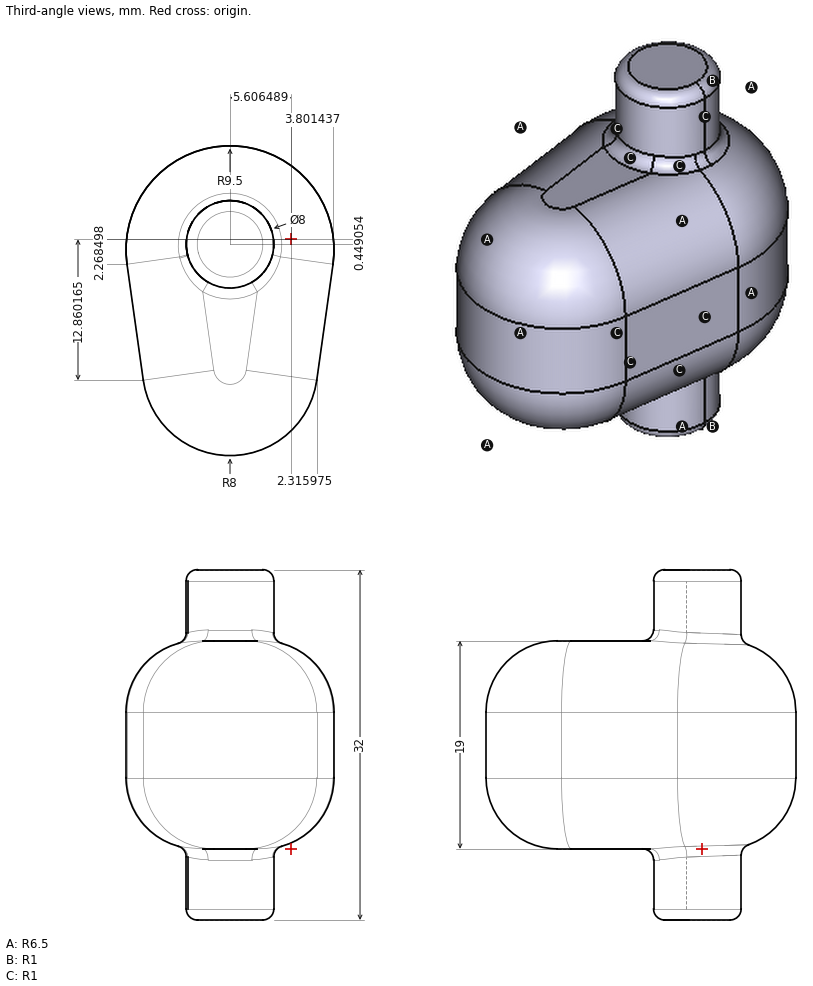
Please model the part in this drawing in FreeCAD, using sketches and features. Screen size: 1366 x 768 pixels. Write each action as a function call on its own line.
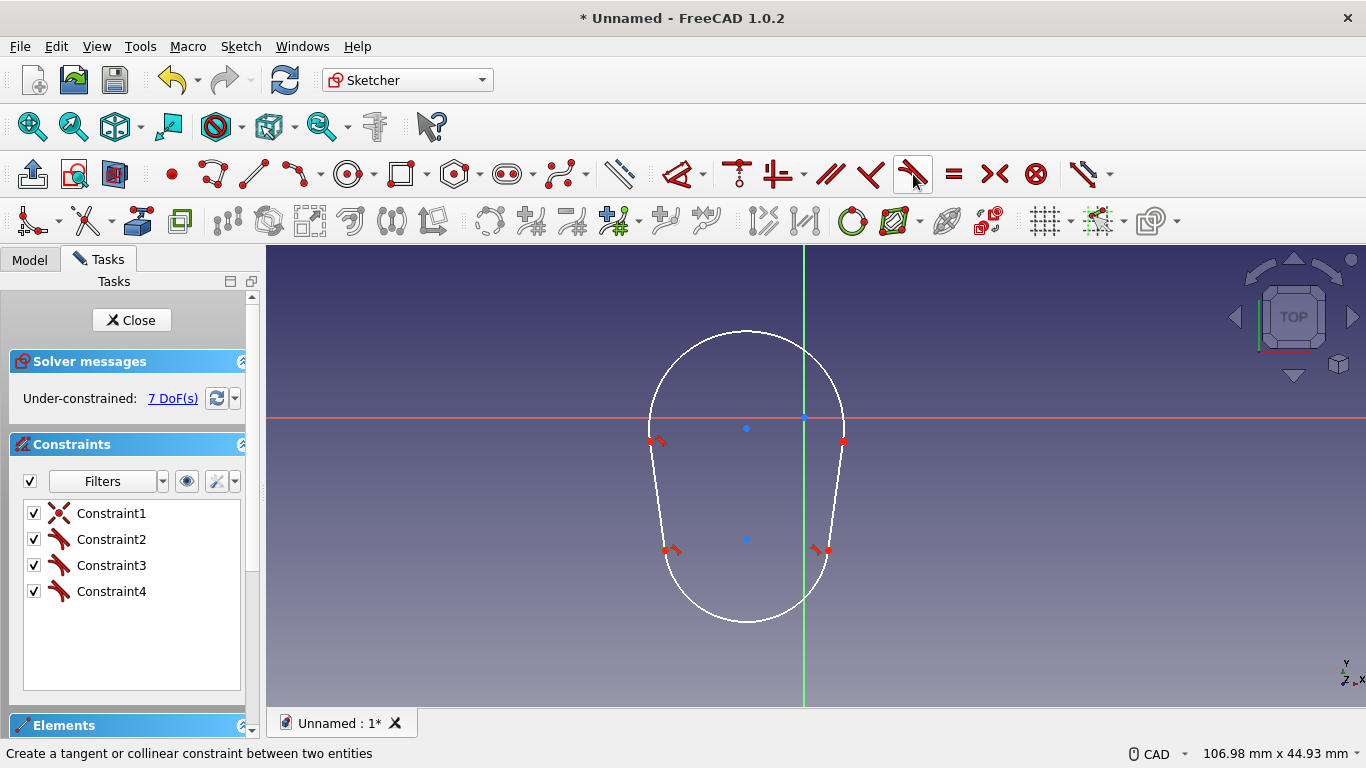
click(832, 518)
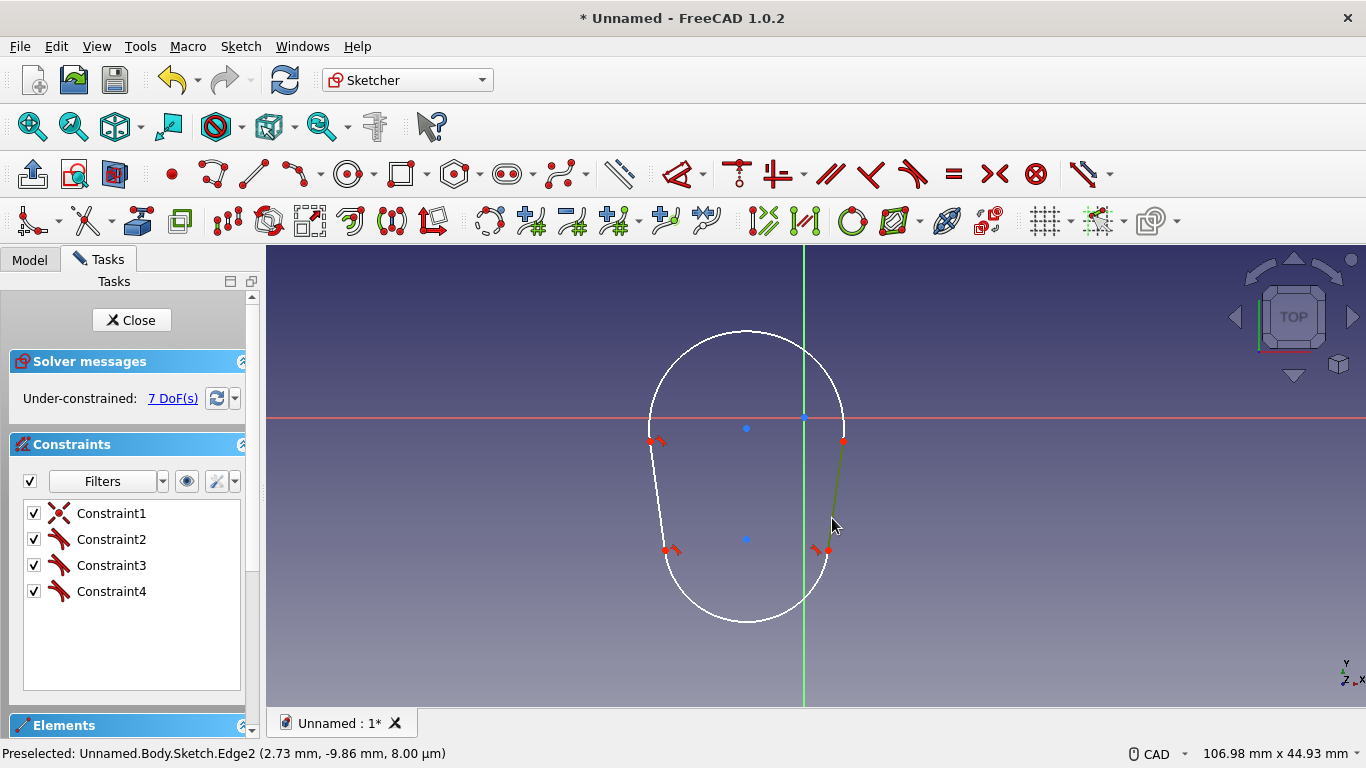
click(808, 353)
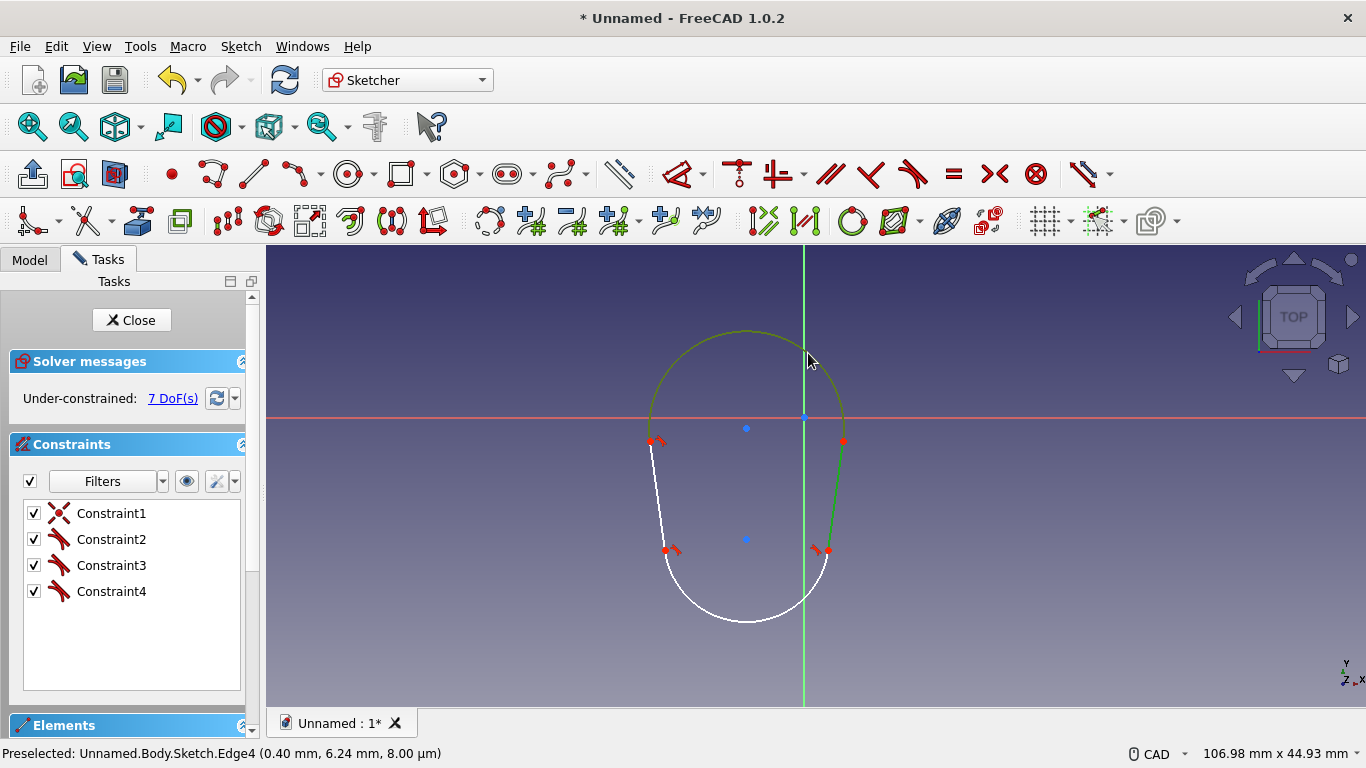
key(t)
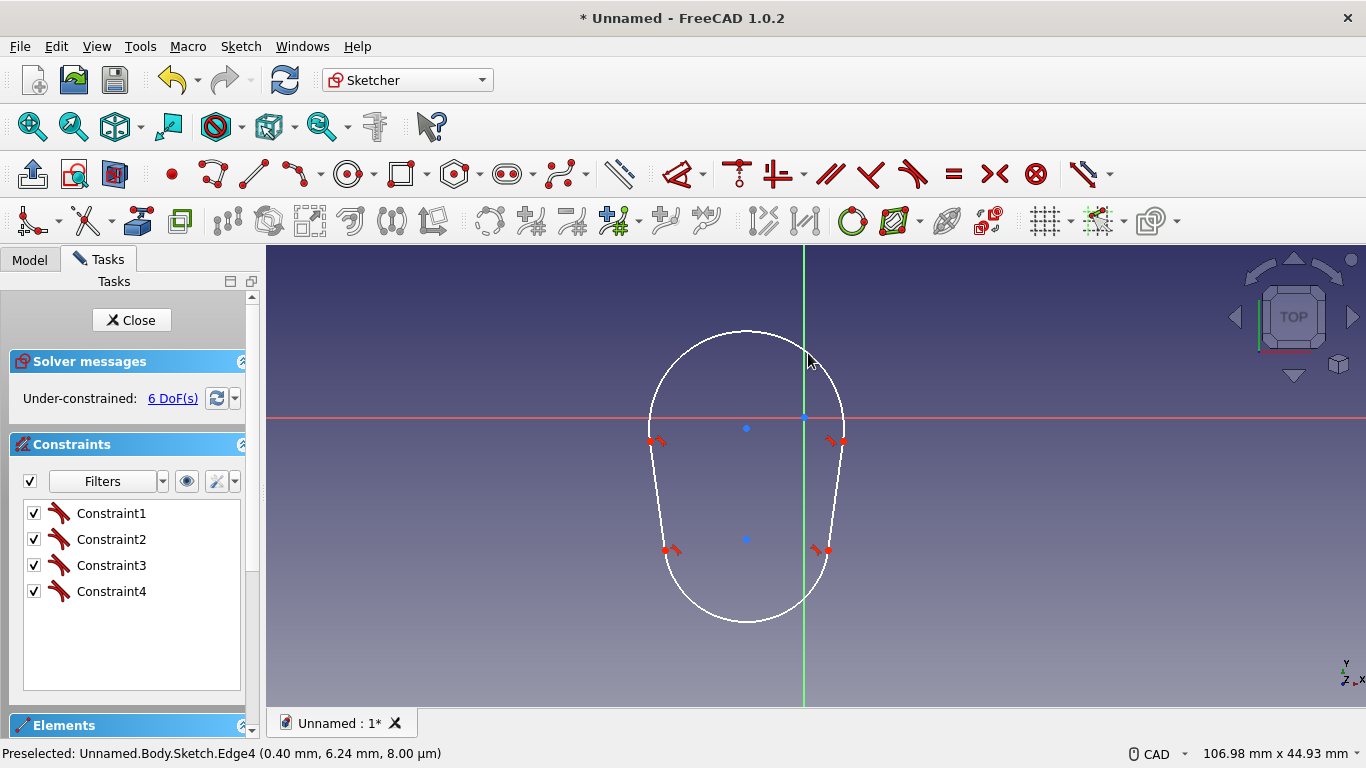
click(702, 609)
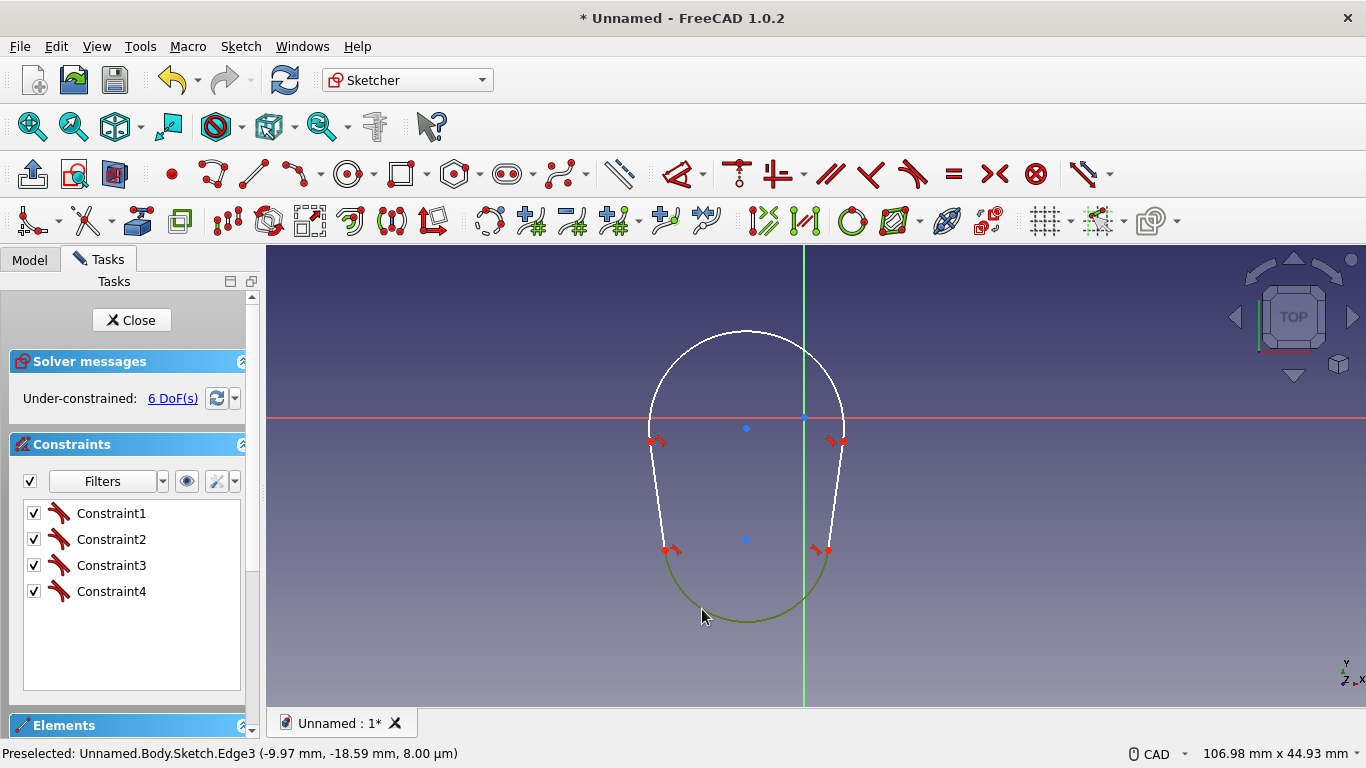
key(k)
key(r)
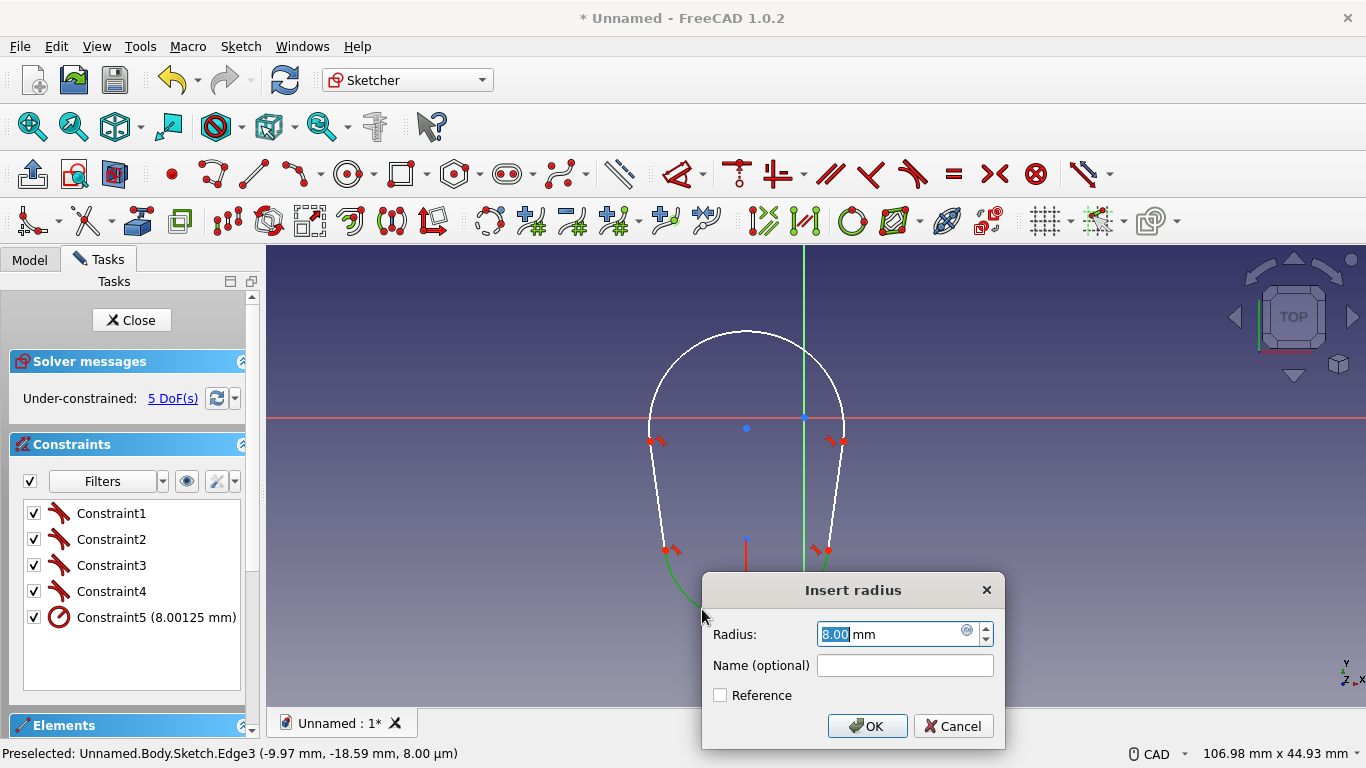
text(8)
key(Return)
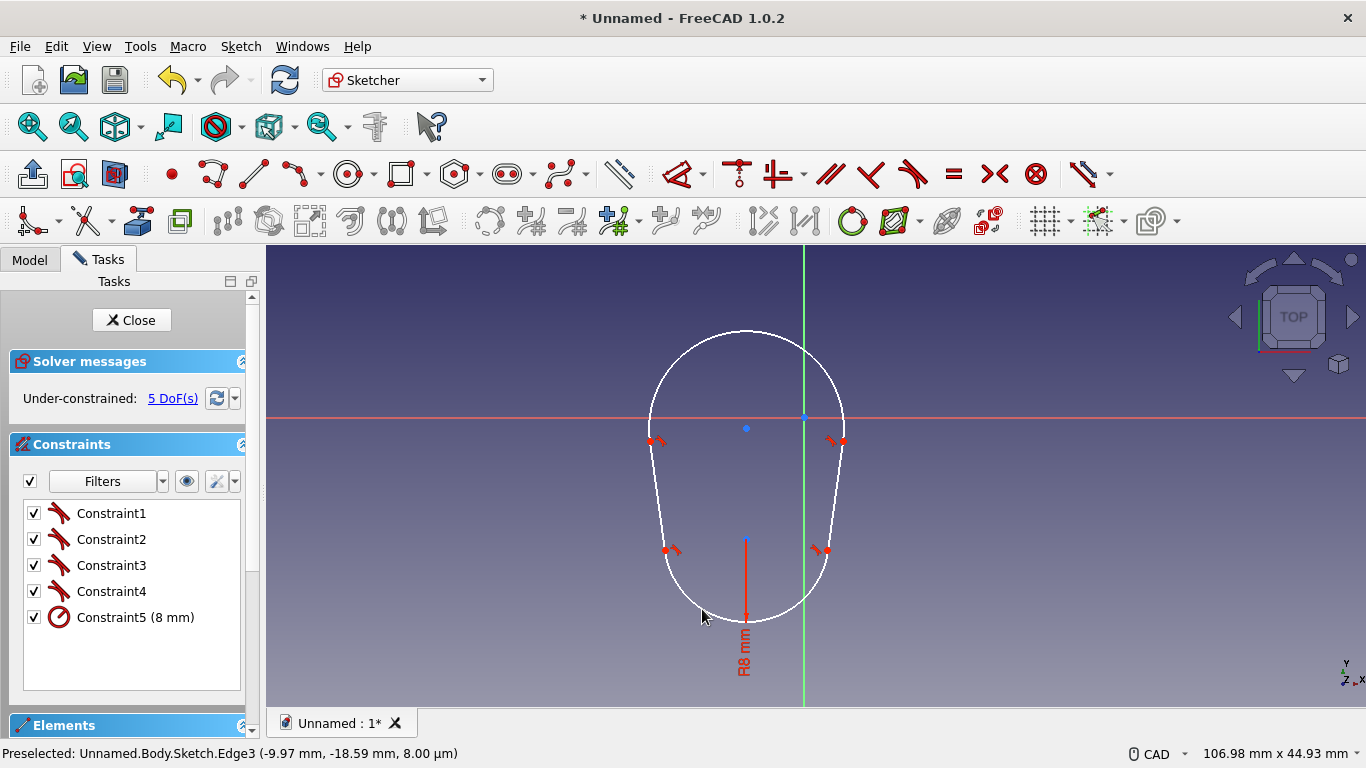
click(808, 353)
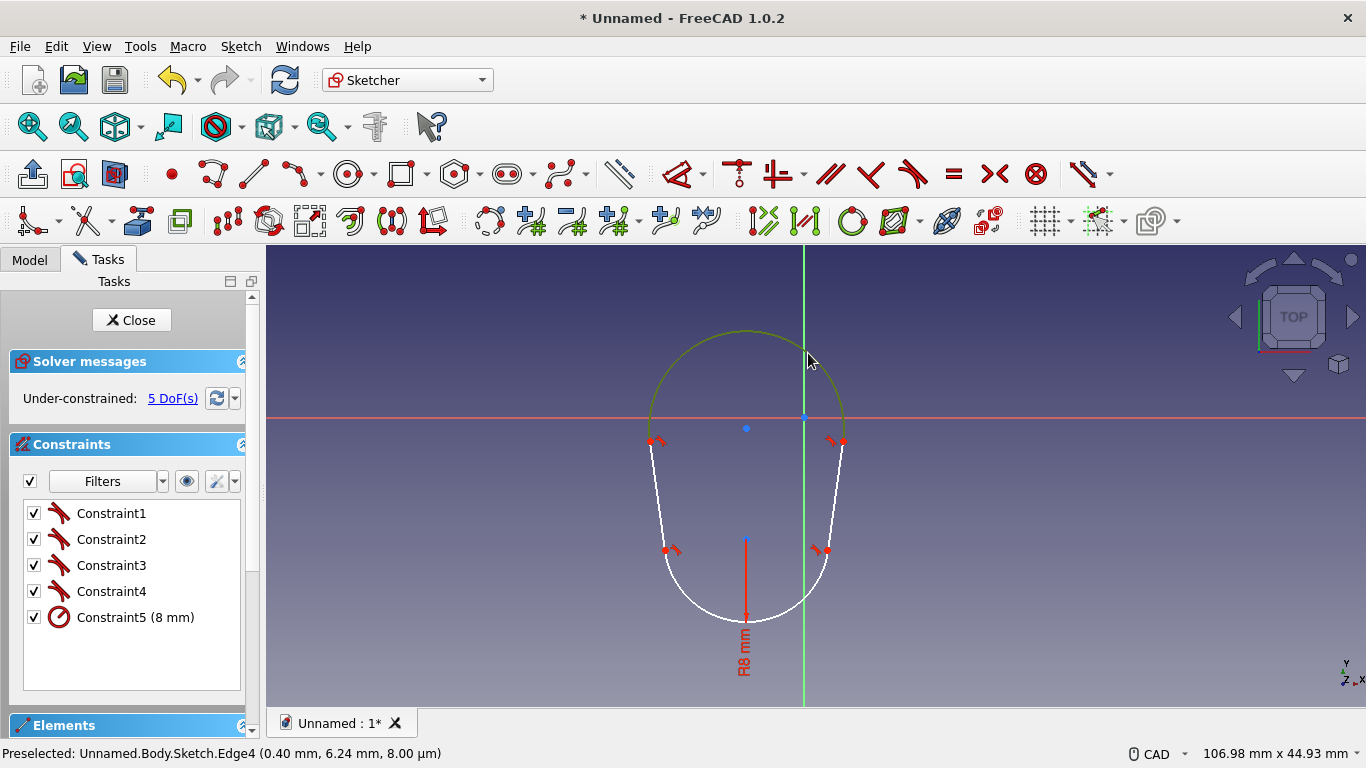
key(k)
key(r)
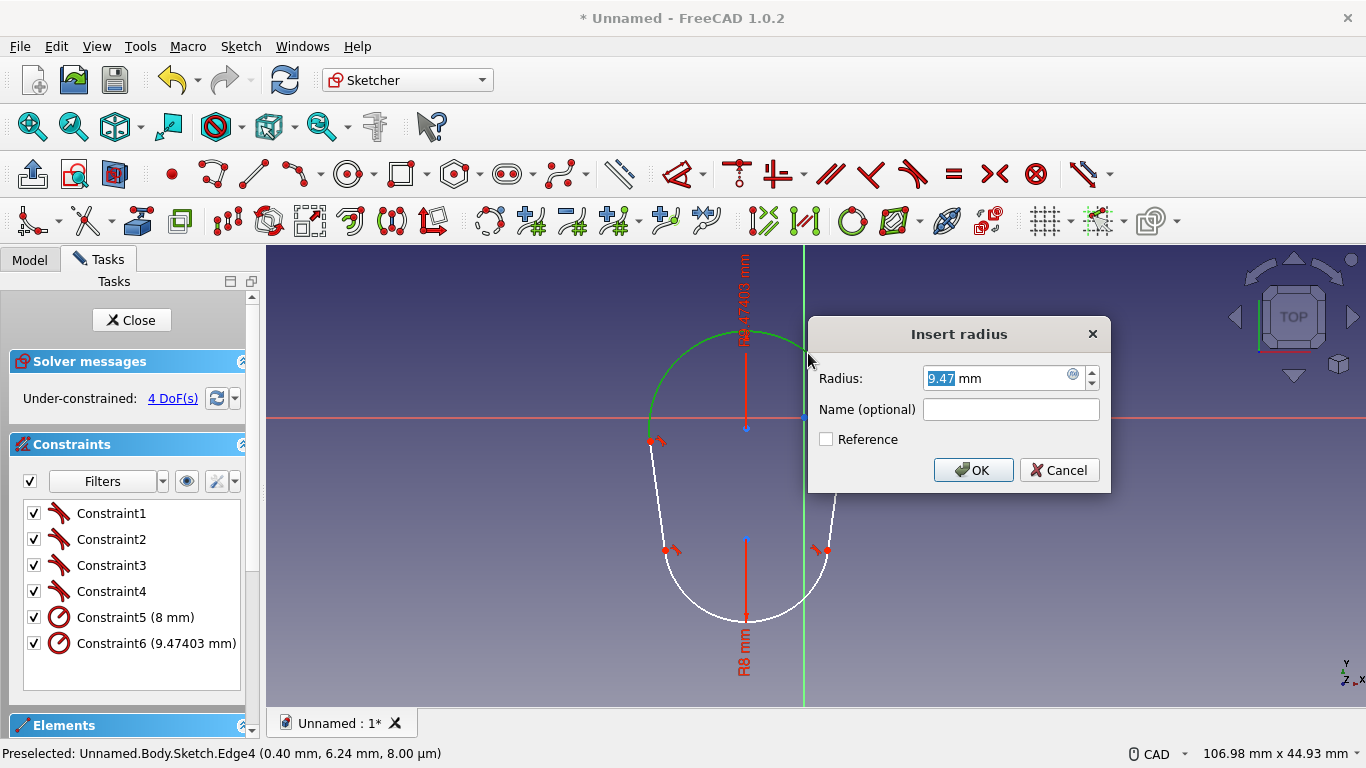
text(9.5)
key(Return)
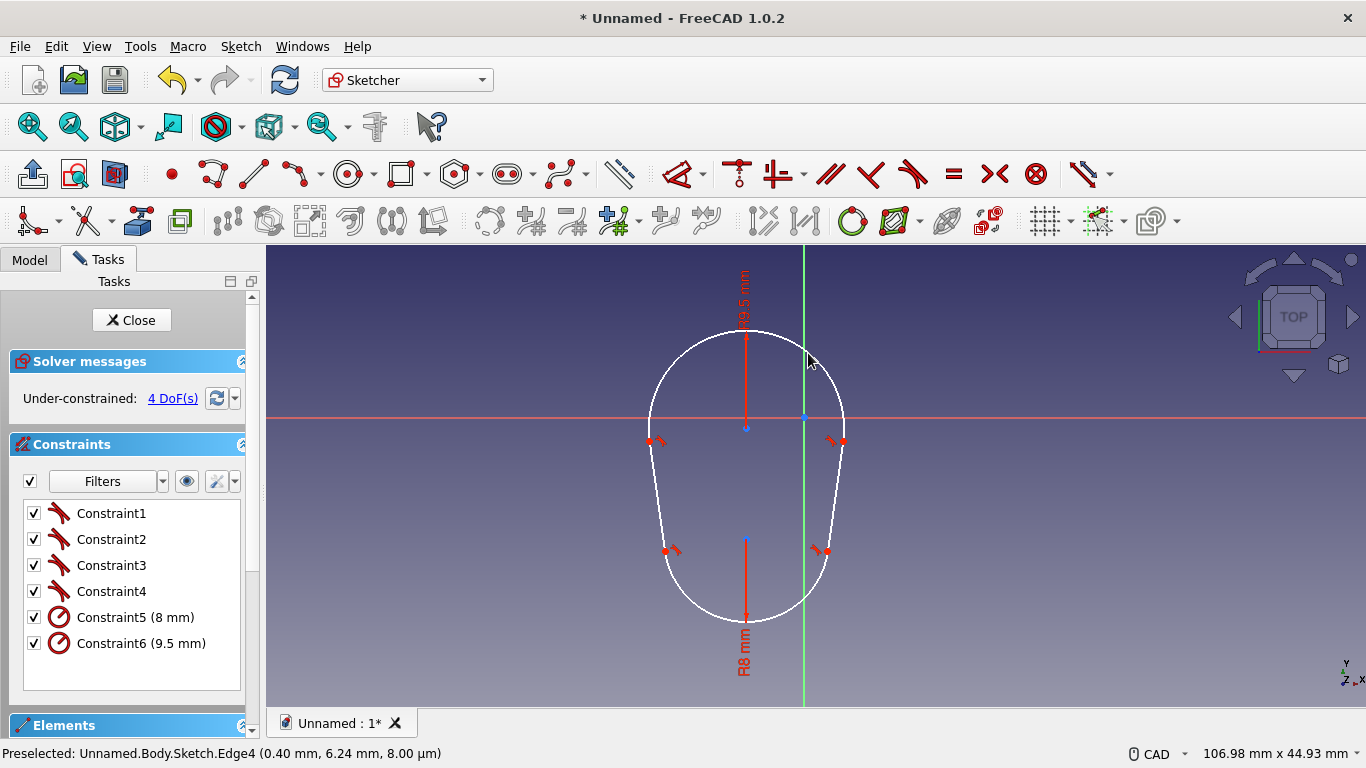
scroll(650, 442, up, 3)